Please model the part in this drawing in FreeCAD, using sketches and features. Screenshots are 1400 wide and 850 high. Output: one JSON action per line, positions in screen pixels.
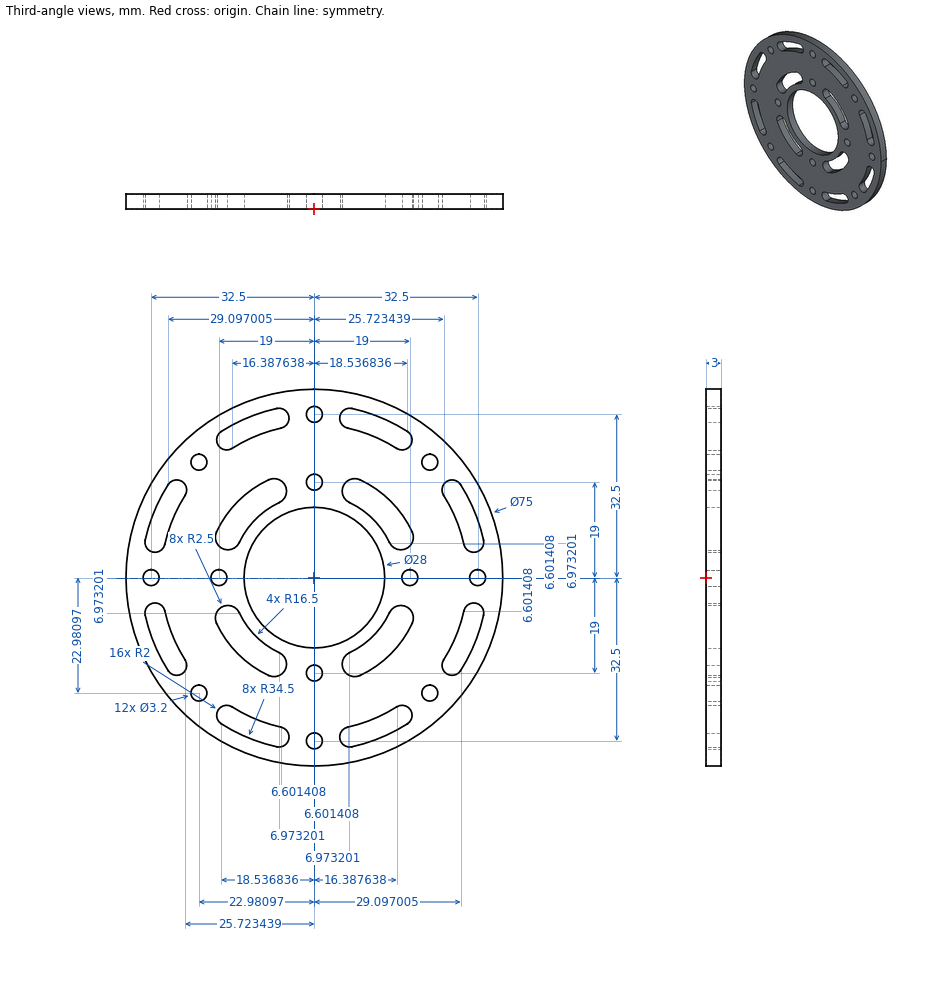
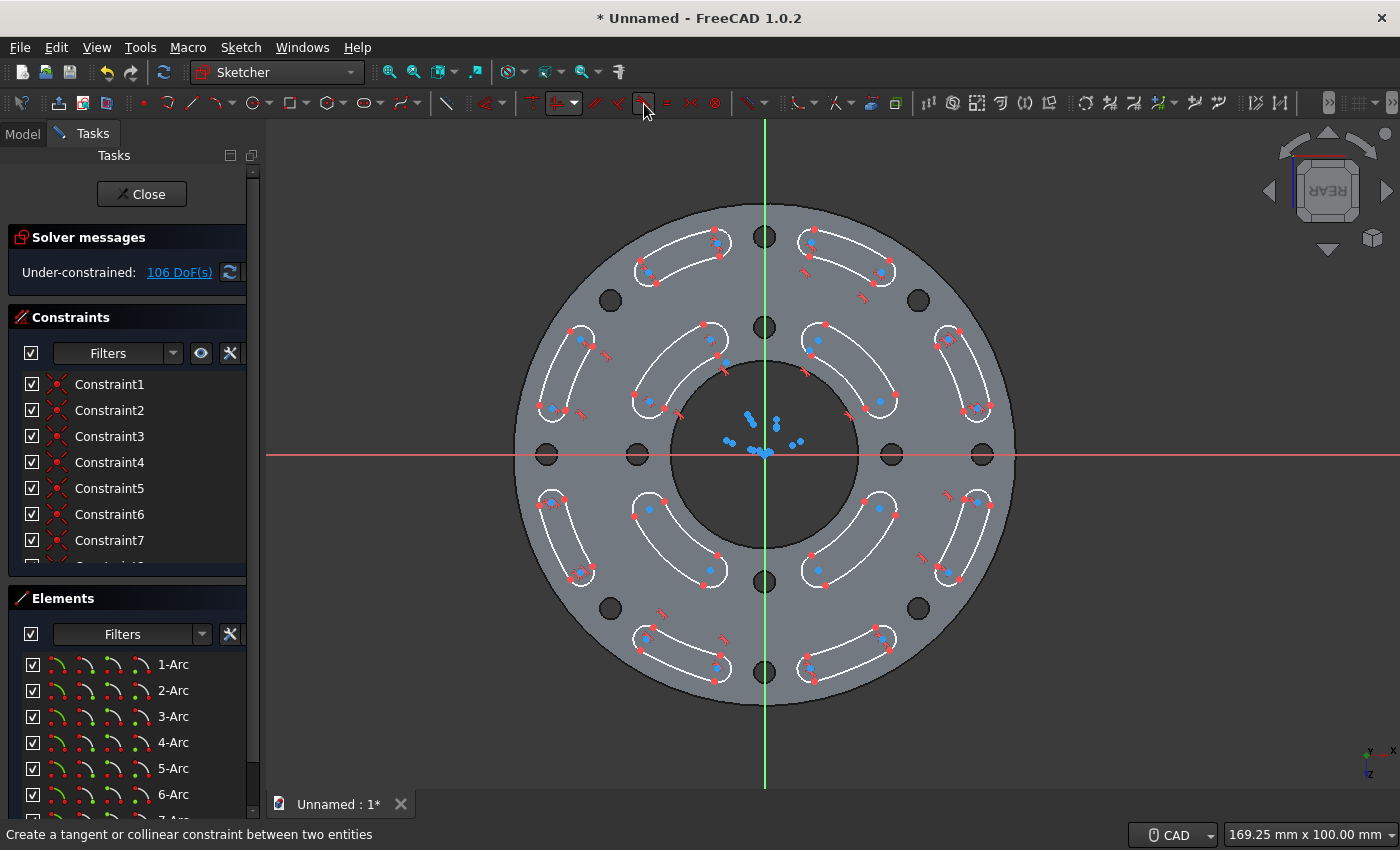
{"action": "left_click", "coordinate": [877, 417]}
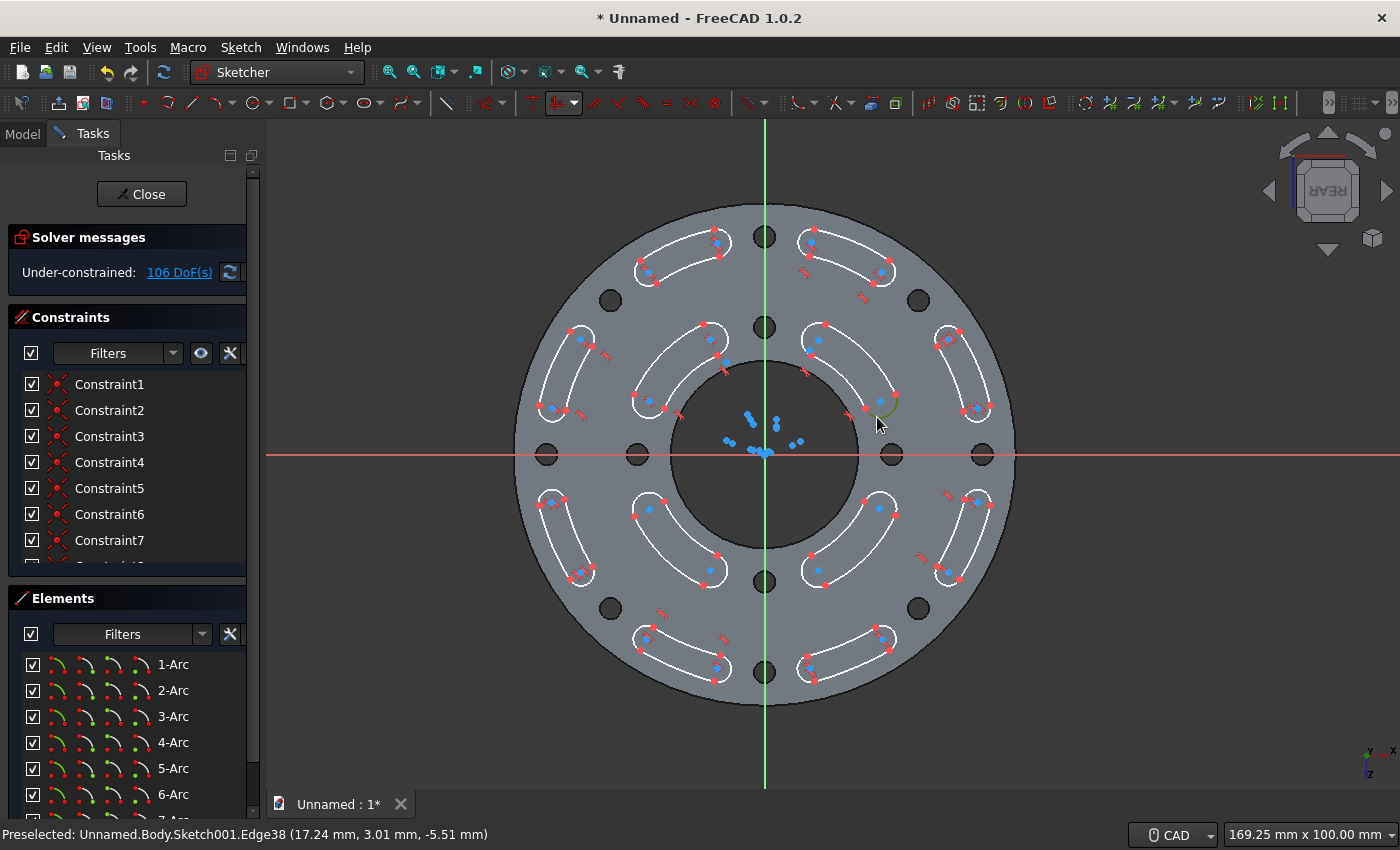
{"action": "left_click", "coordinate": [880, 368]}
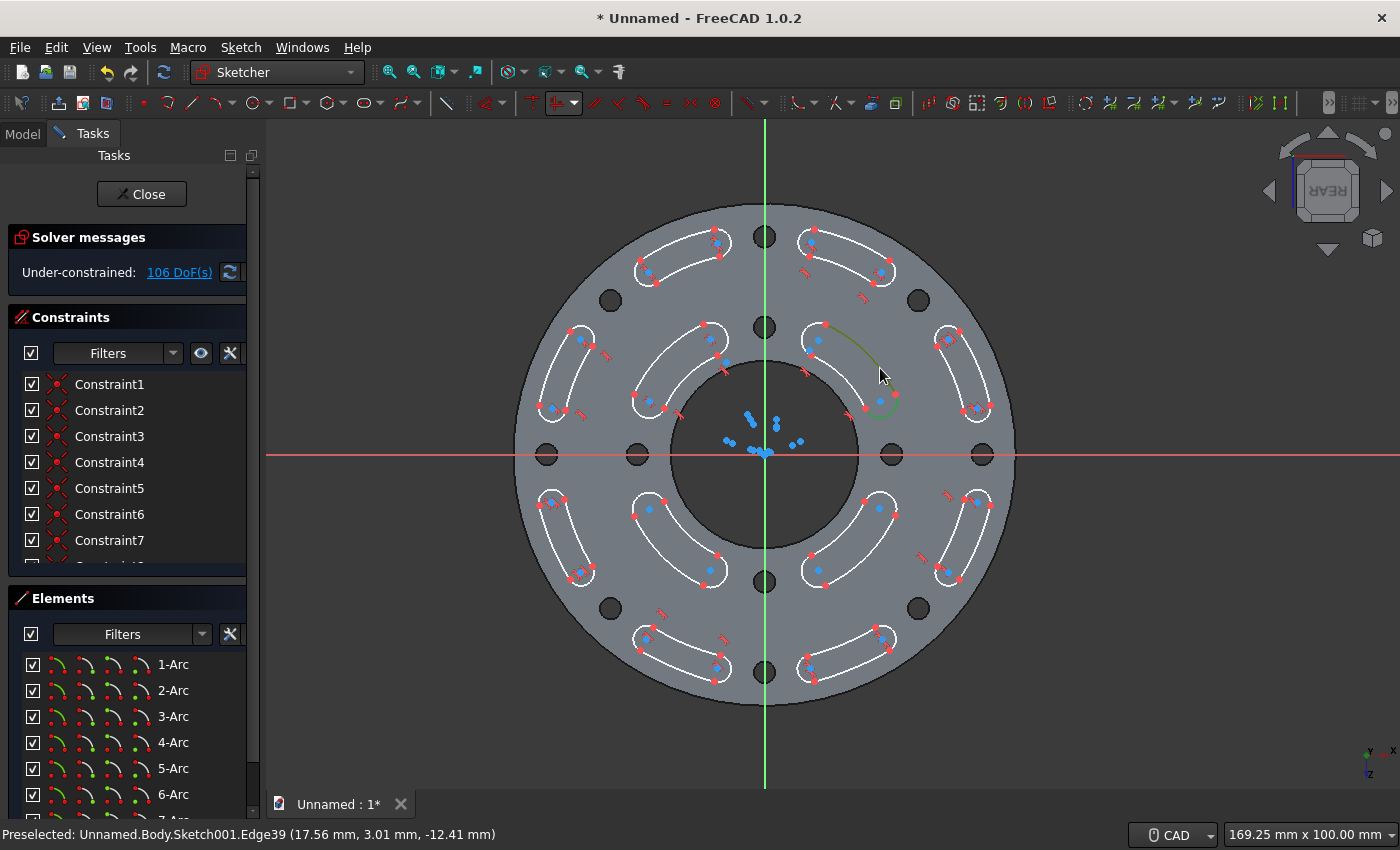
{"action": "left_click", "coordinate": [644, 104]}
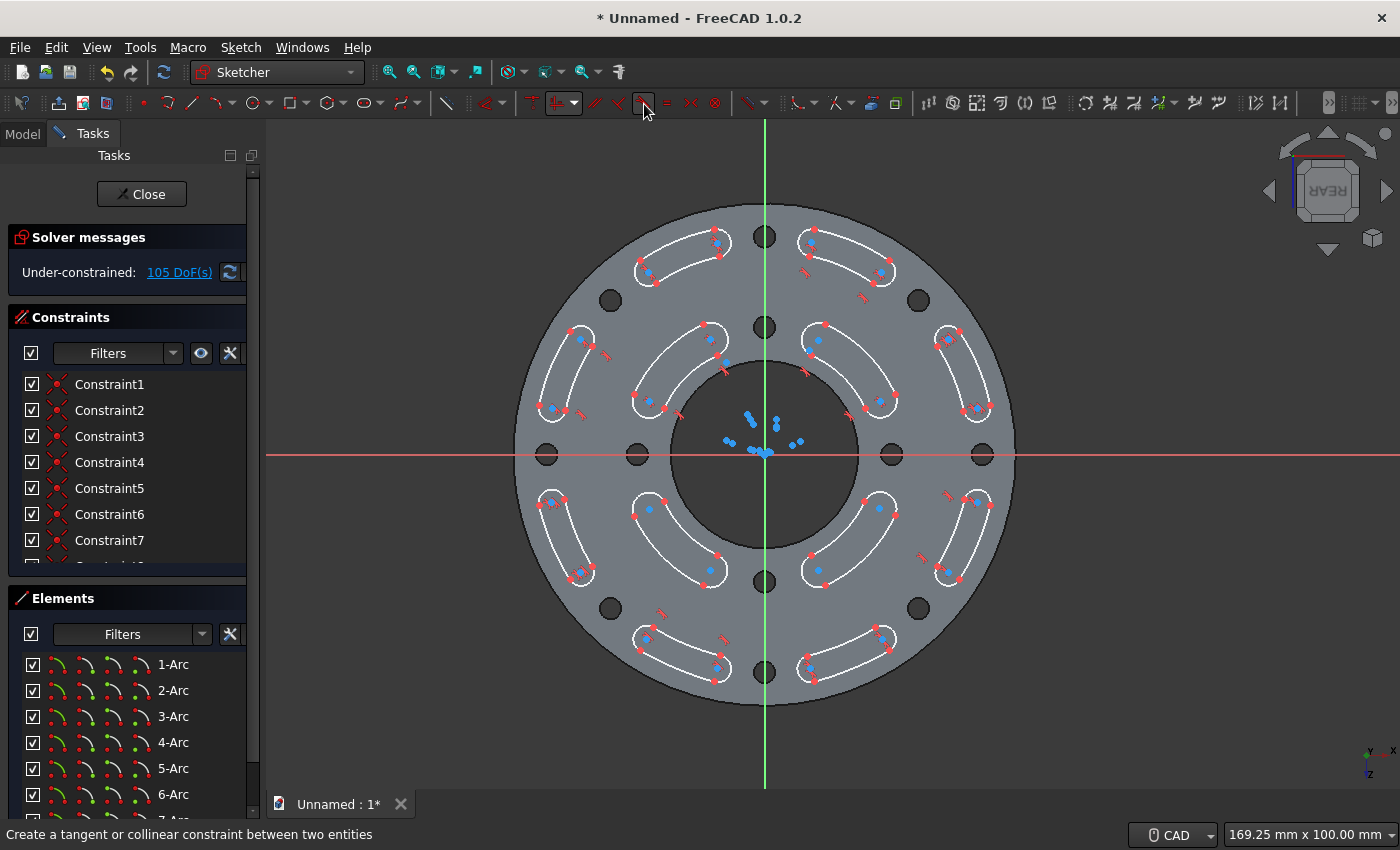
{"action": "left_click", "coordinate": [880, 368]}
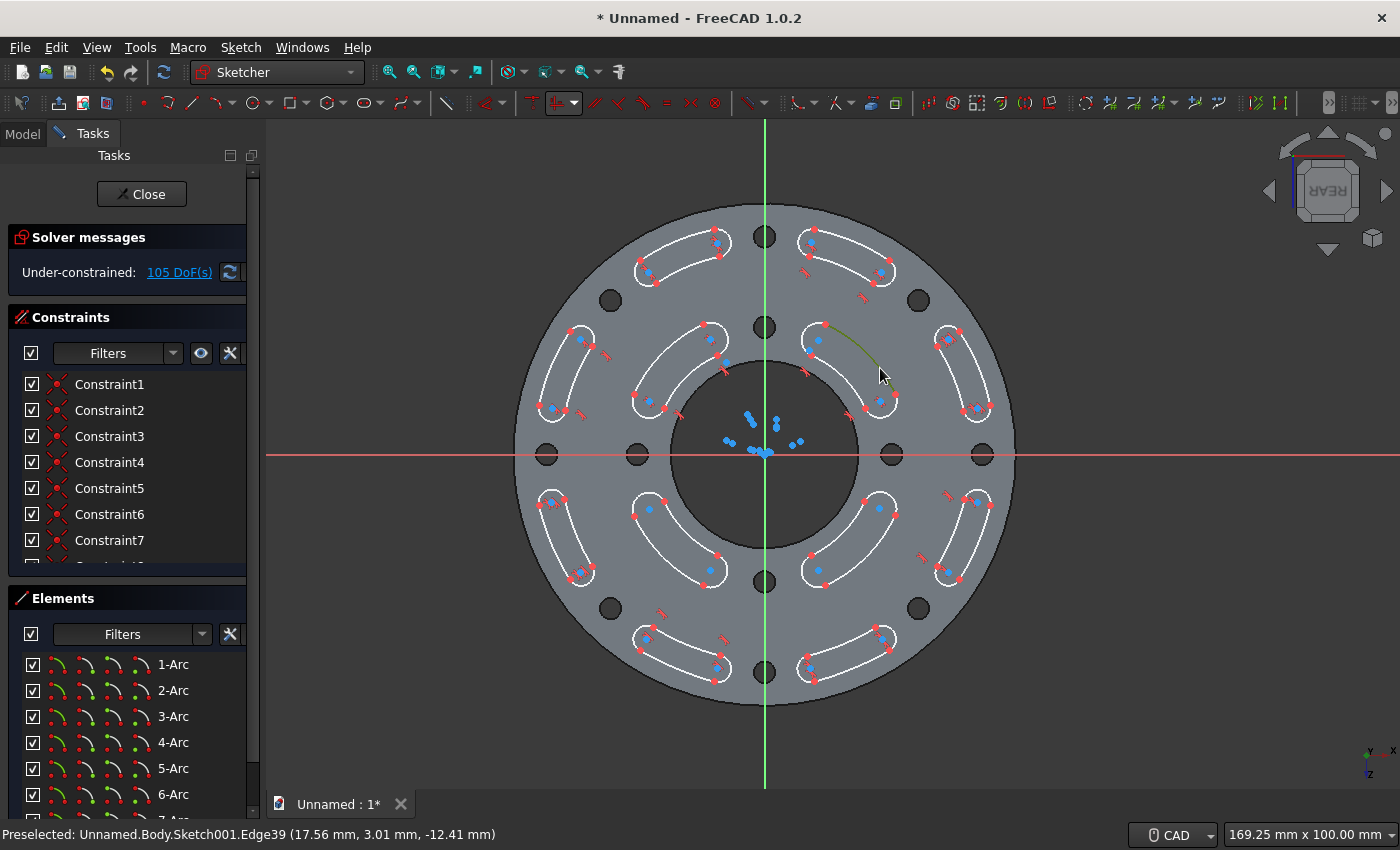
{"action": "left_click", "coordinate": [810, 325]}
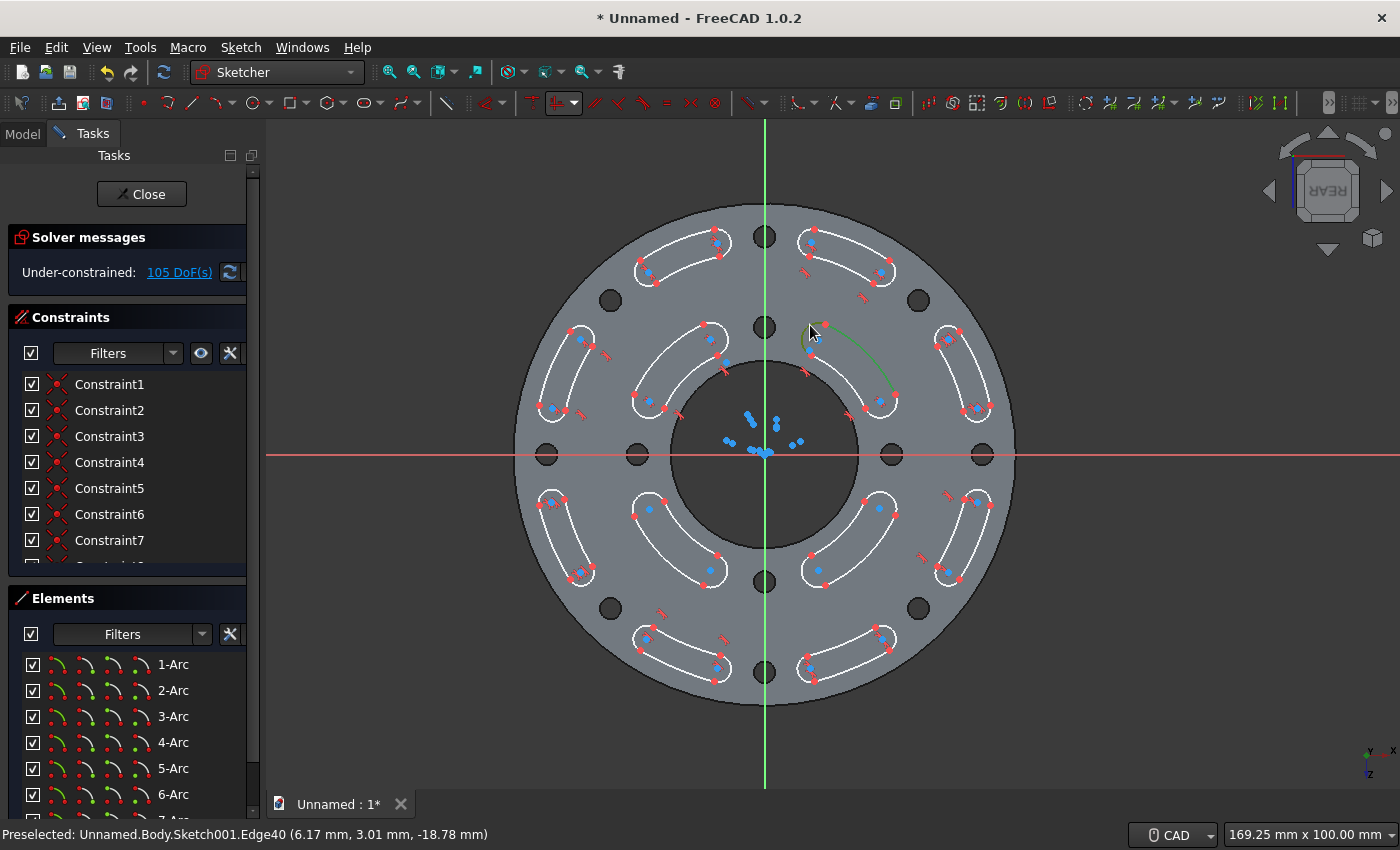
{"action": "left_click", "coordinate": [644, 104]}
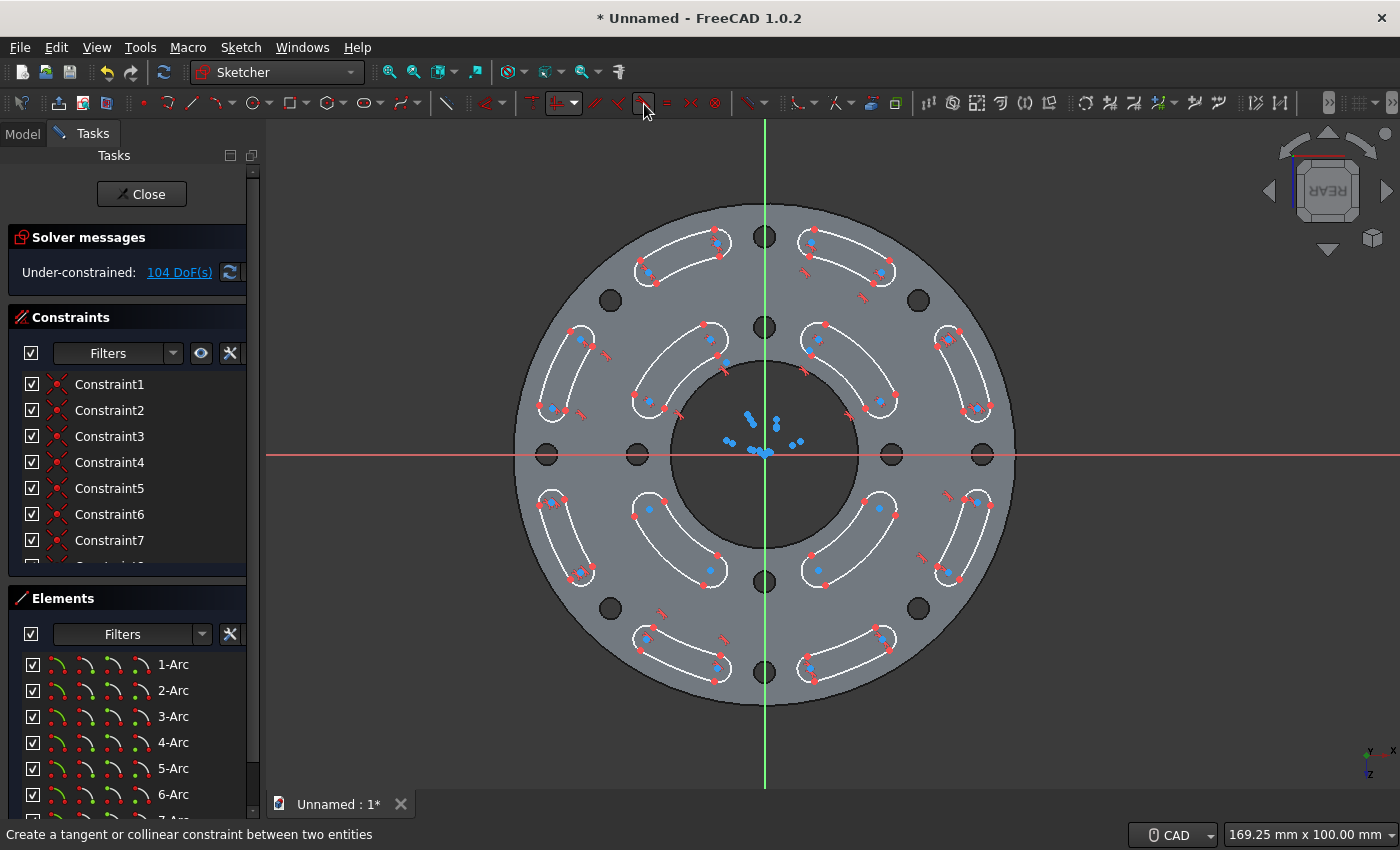
{"action": "left_click", "coordinate": [831, 543]}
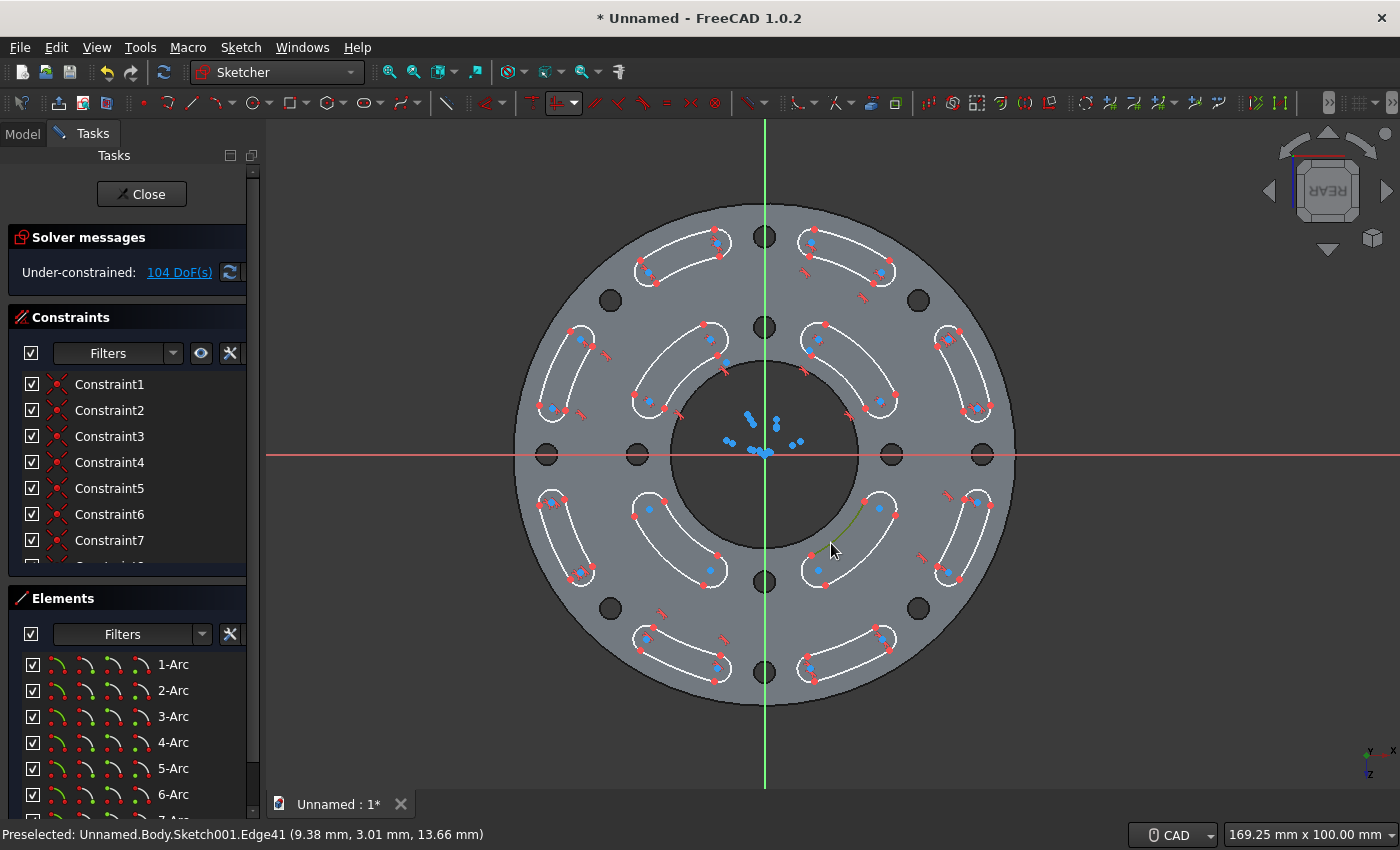
{"action": "left_click", "coordinate": [802, 568]}